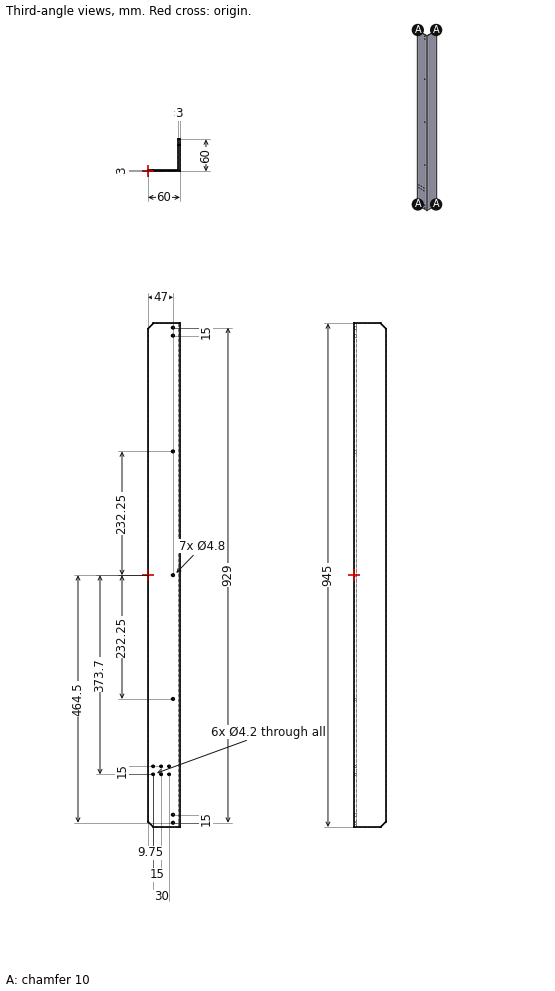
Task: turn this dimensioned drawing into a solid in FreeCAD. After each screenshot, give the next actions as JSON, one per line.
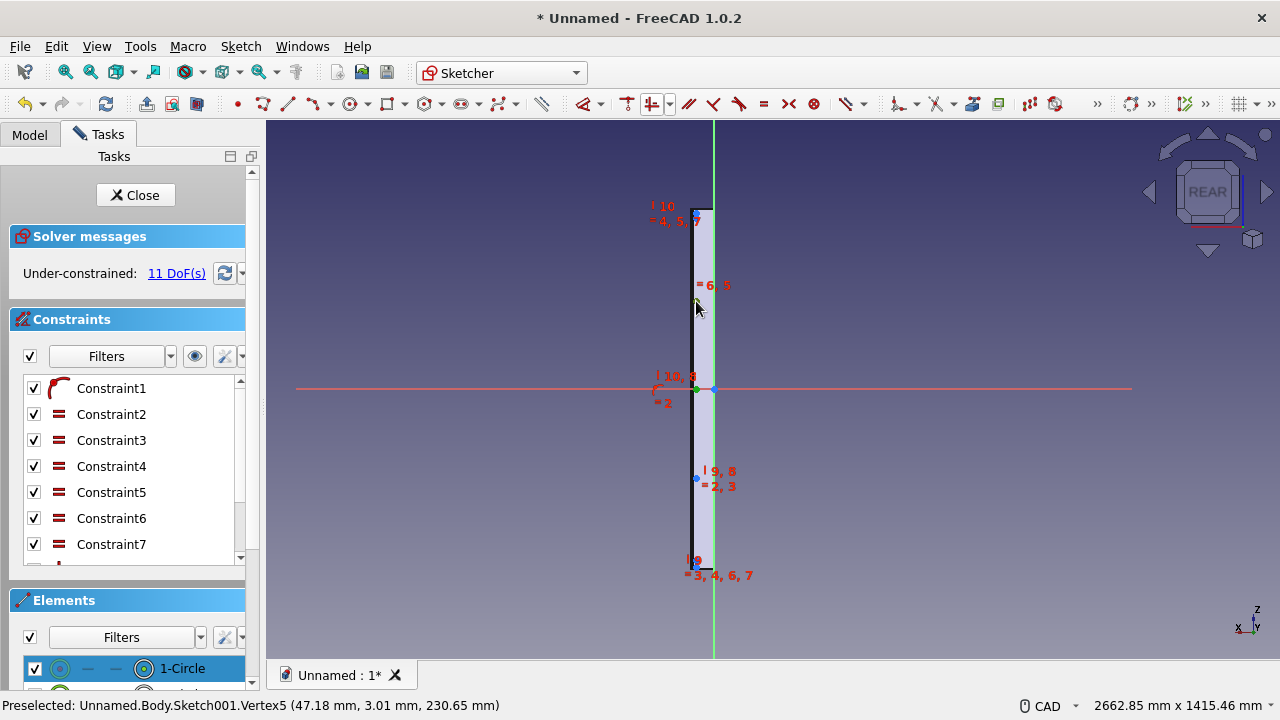
{"action": "key", "text": "v"}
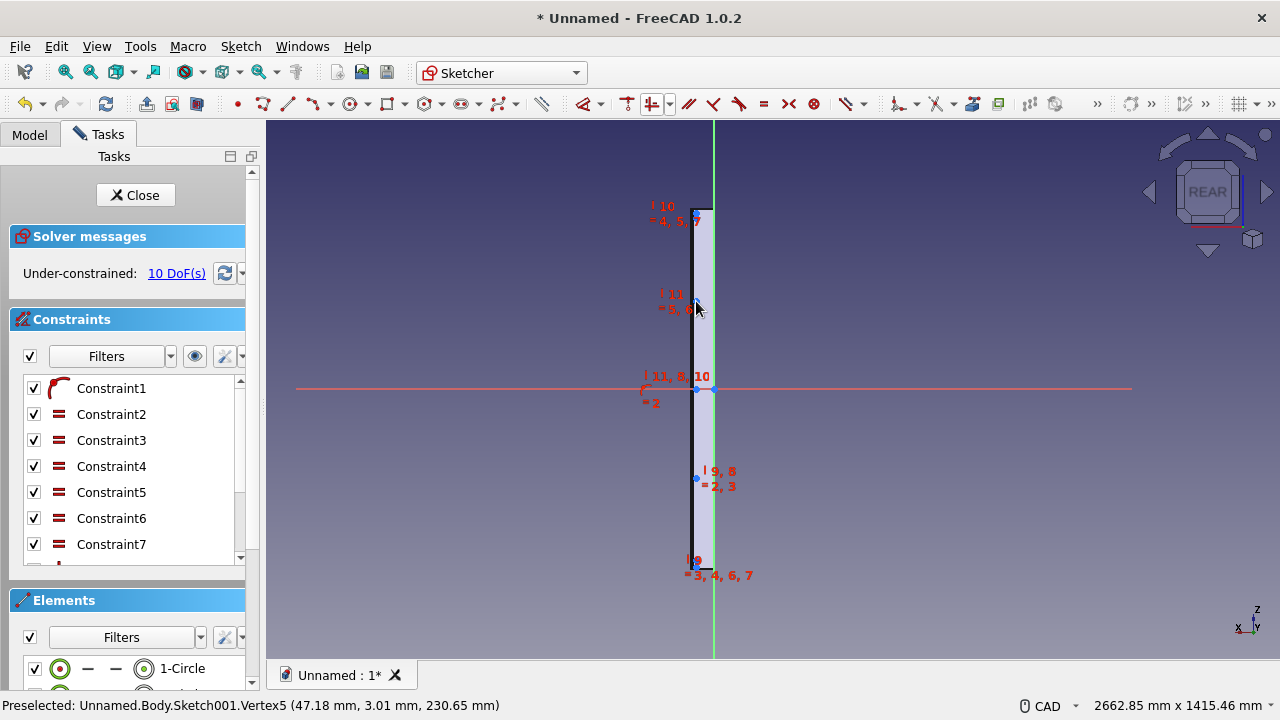
{"action": "scroll", "coordinate": [696, 567], "scroll_direction": "up", "scroll_amount": 3}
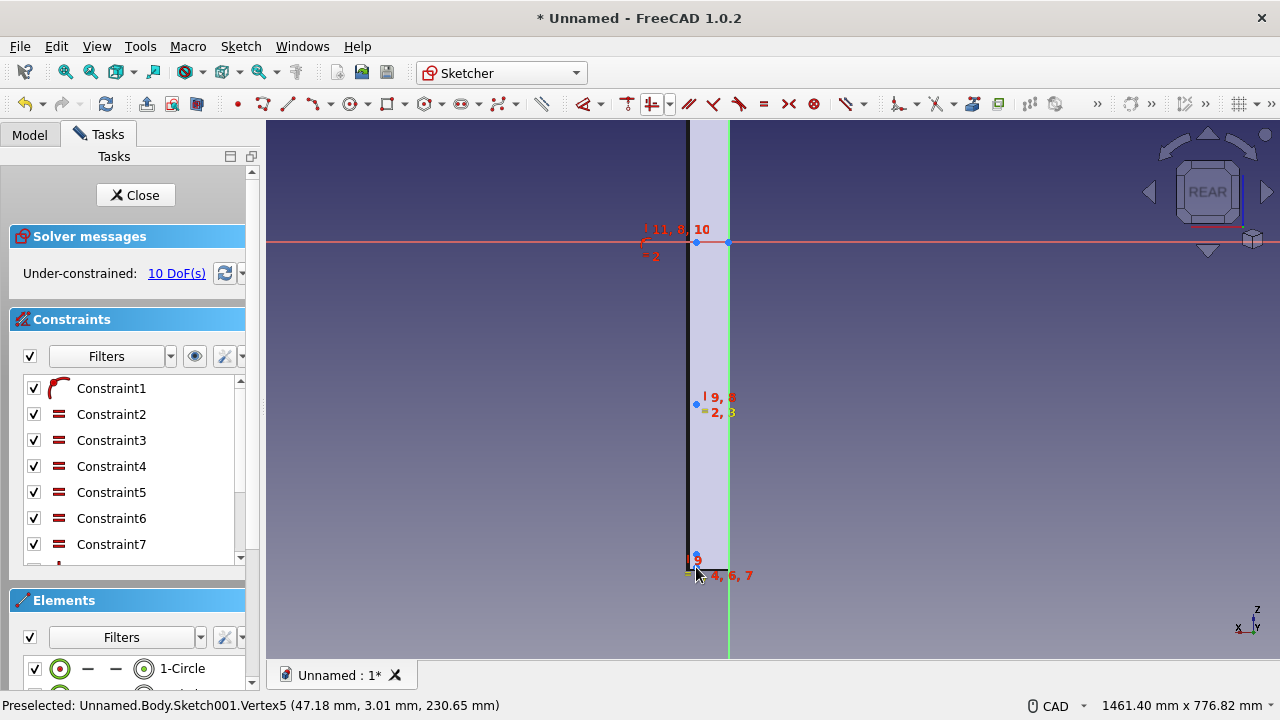
{"action": "scroll", "coordinate": [696, 567], "scroll_direction": "up", "scroll_amount": 4}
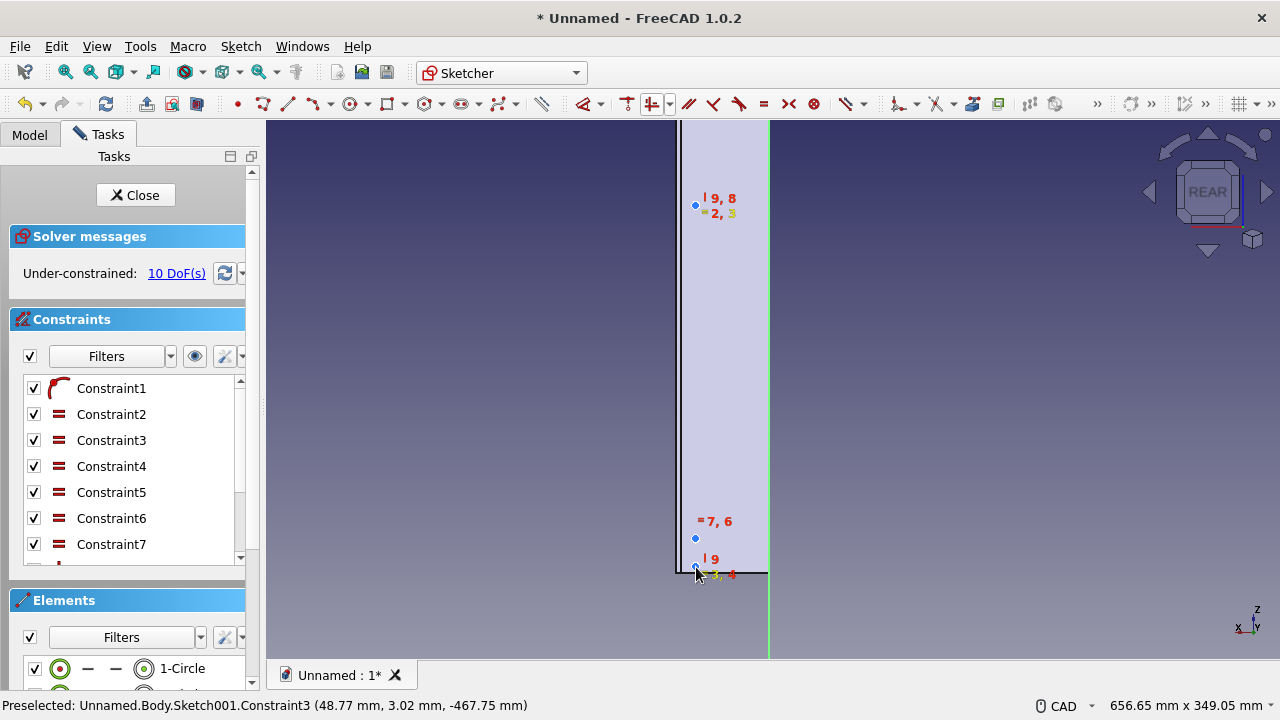
{"action": "left_click", "coordinate": [696, 566]}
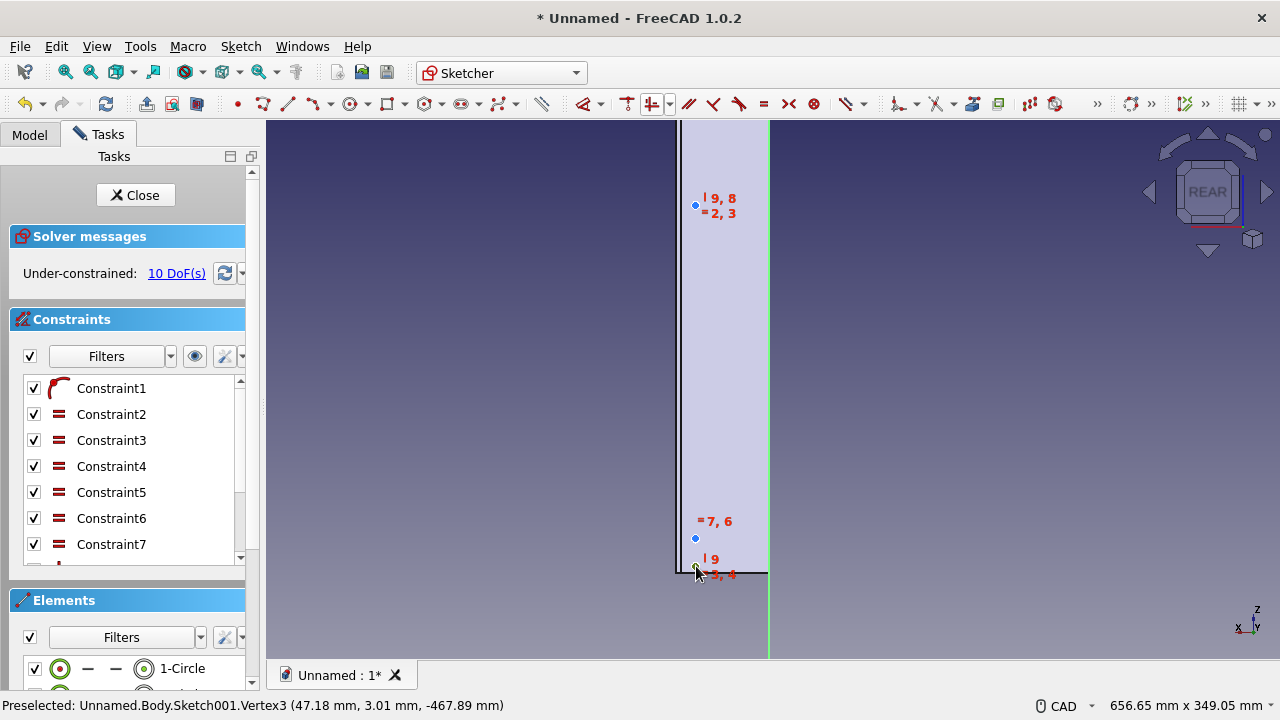
{"action": "left_click", "coordinate": [696, 539]}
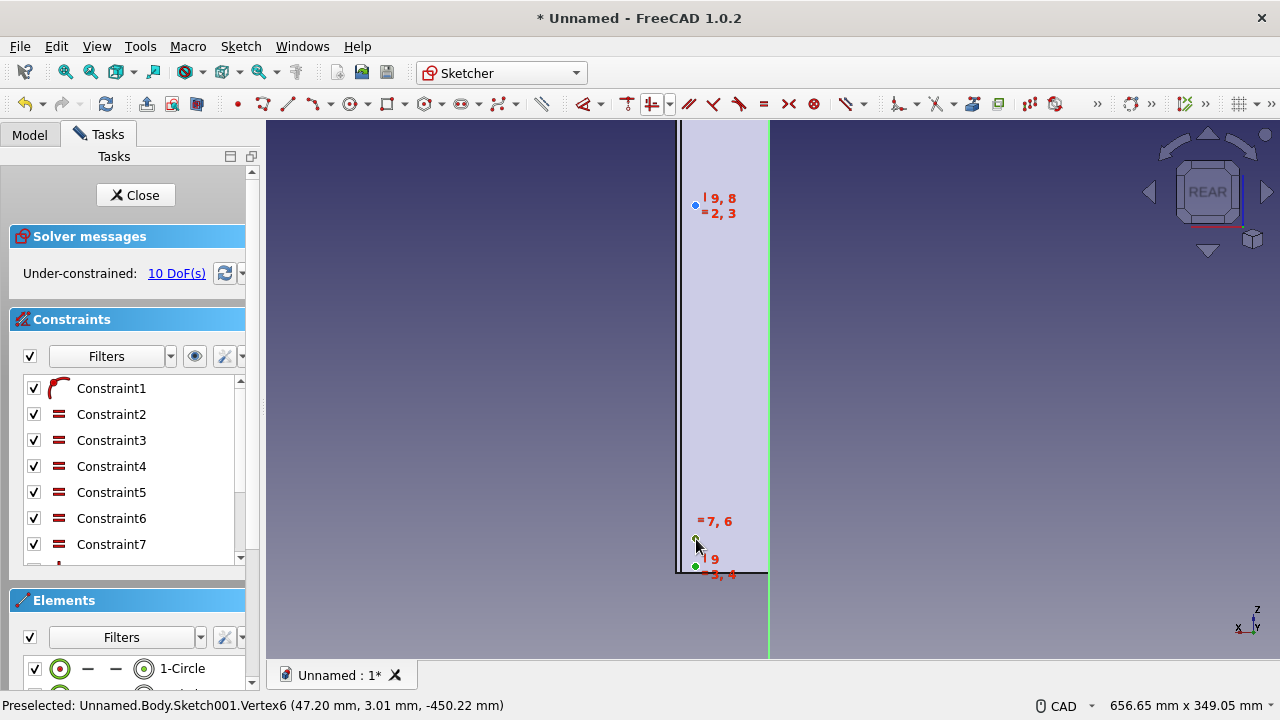
{"action": "key", "text": "v"}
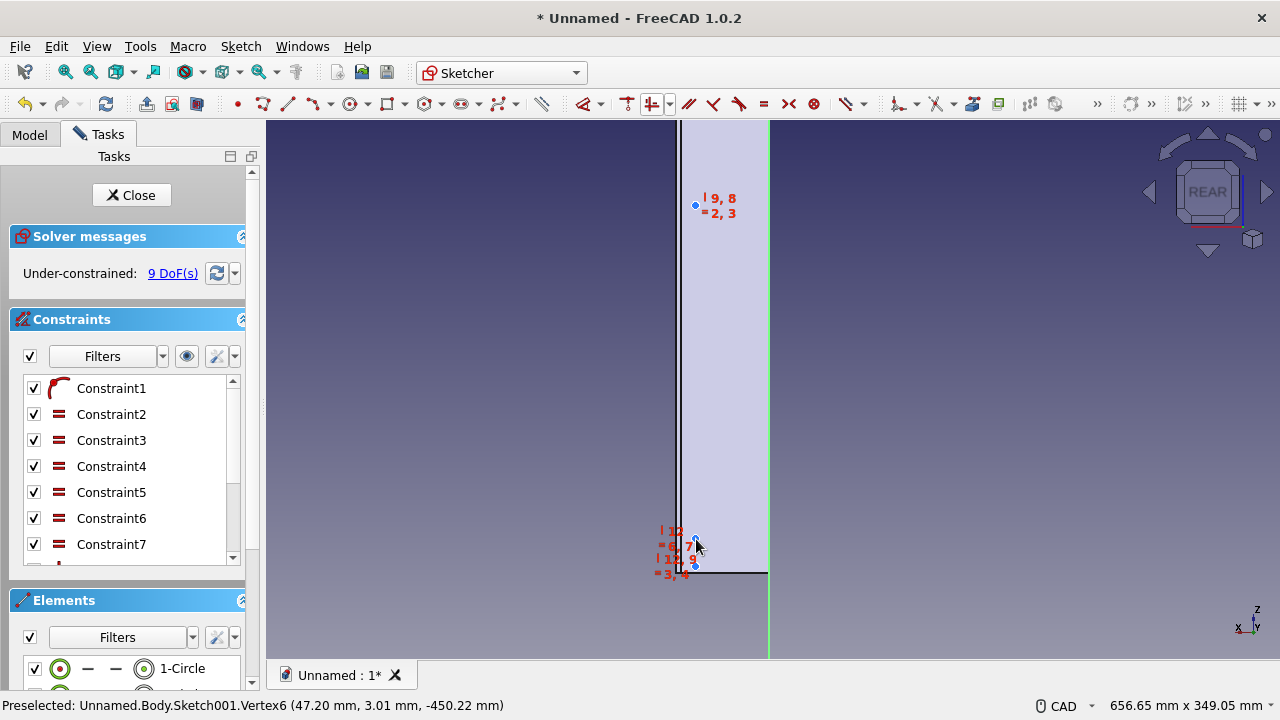
{"action": "scroll", "coordinate": [696, 568], "scroll_direction": "down", "scroll_amount": 7}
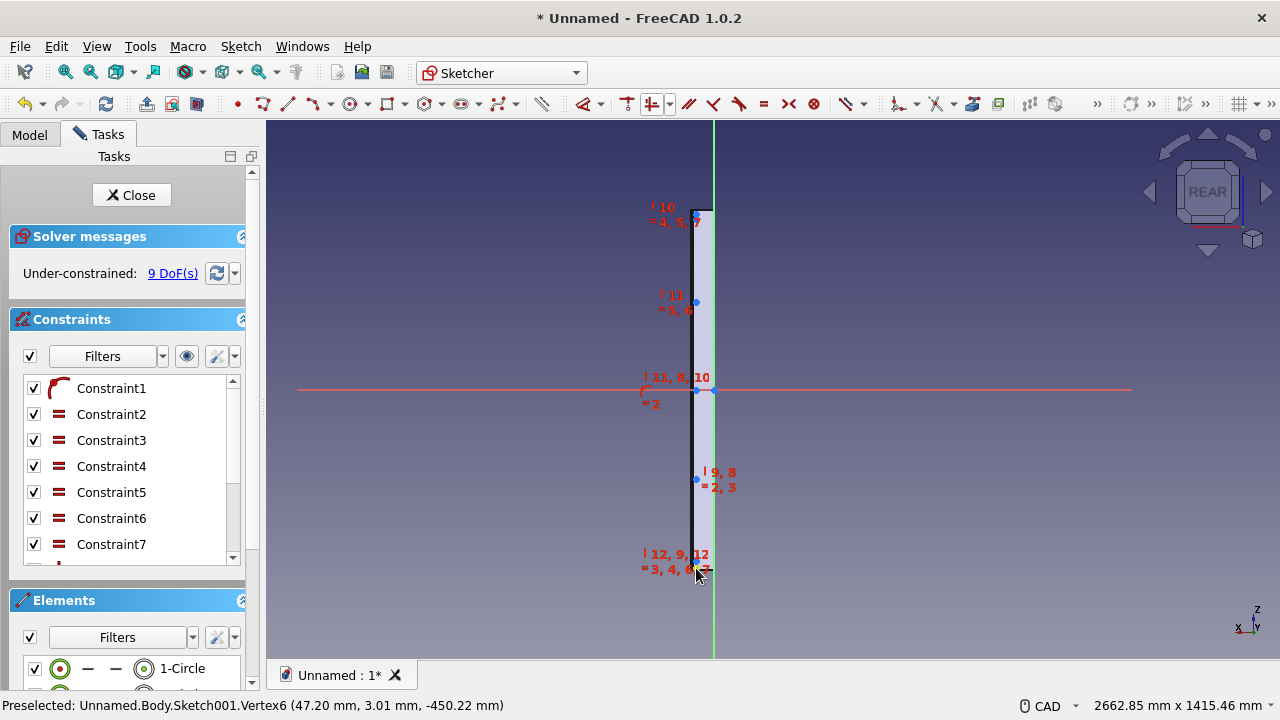
{"action": "scroll", "coordinate": [696, 214], "scroll_direction": "up", "scroll_amount": 5}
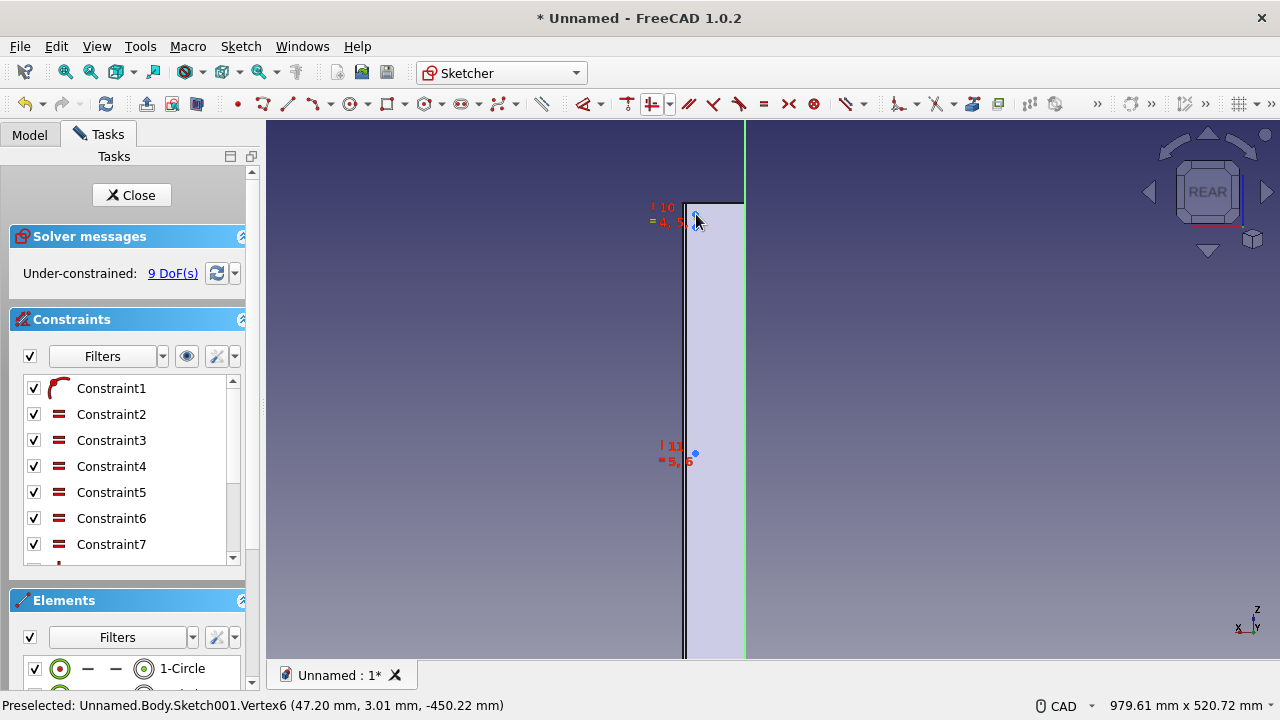
{"action": "scroll", "coordinate": [696, 214], "scroll_direction": "up", "scroll_amount": 4}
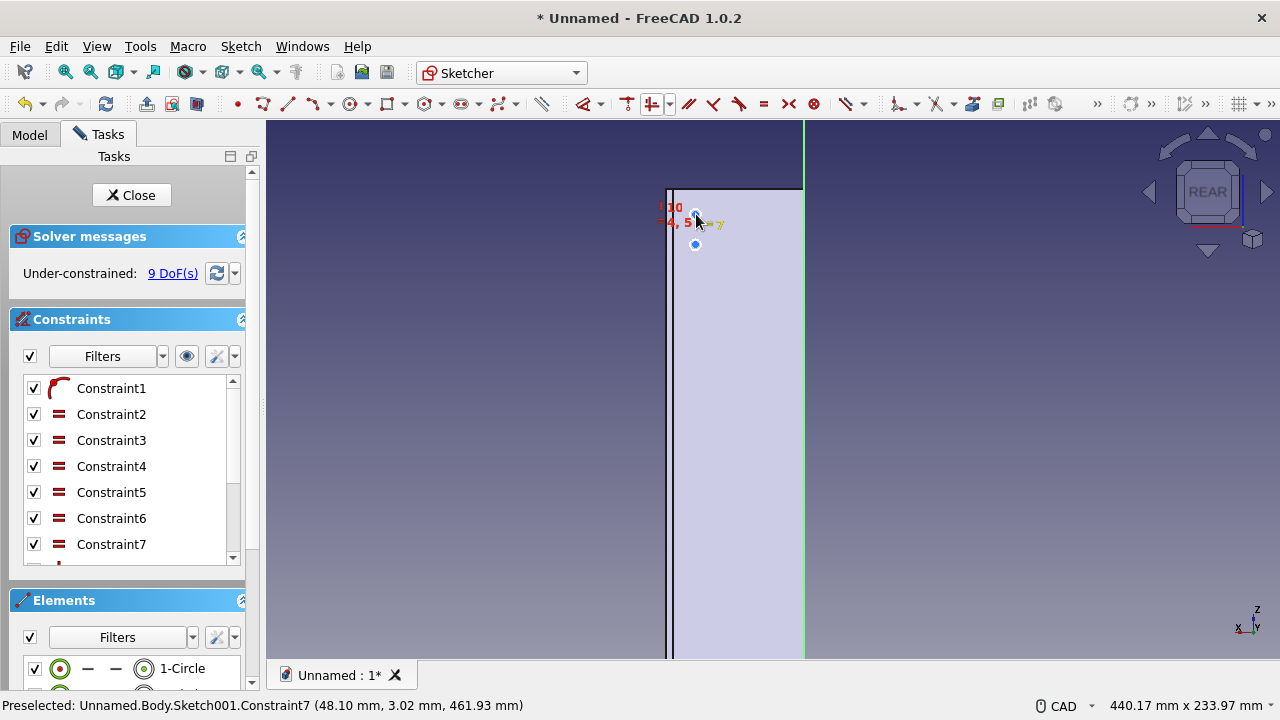
{"action": "left_click", "coordinate": [695, 214]}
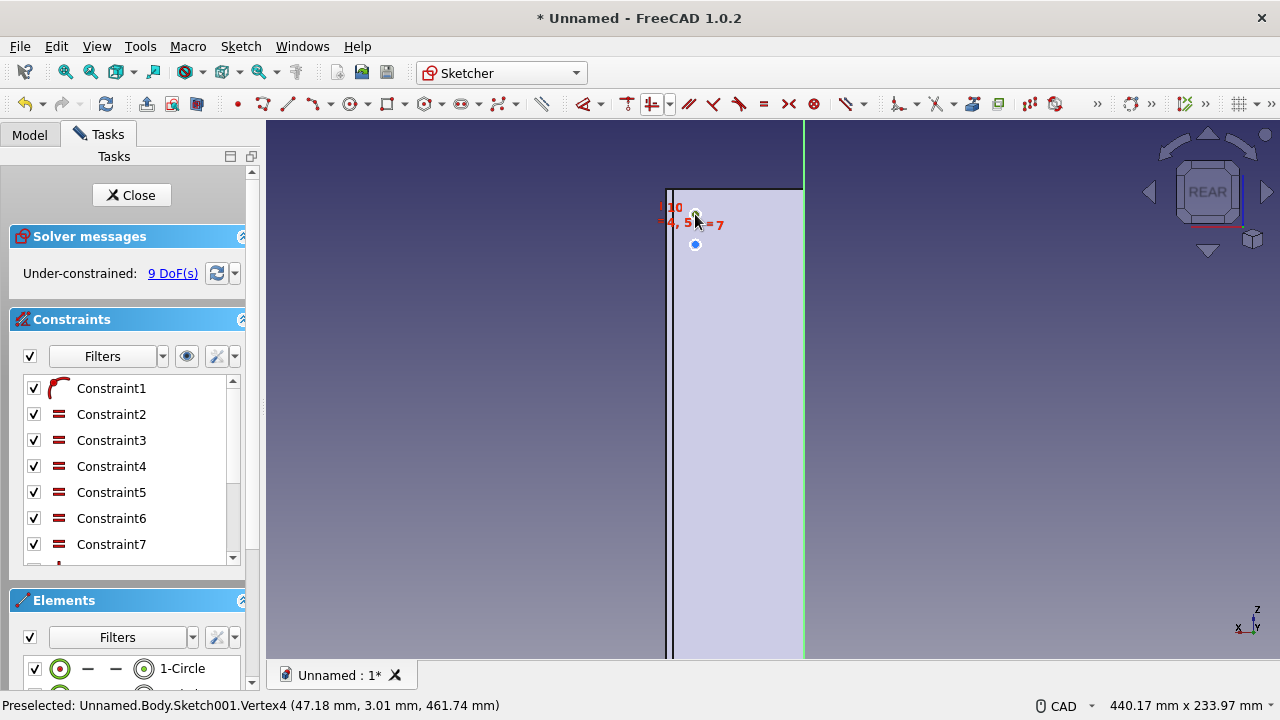
{"action": "left_click", "coordinate": [695, 245]}